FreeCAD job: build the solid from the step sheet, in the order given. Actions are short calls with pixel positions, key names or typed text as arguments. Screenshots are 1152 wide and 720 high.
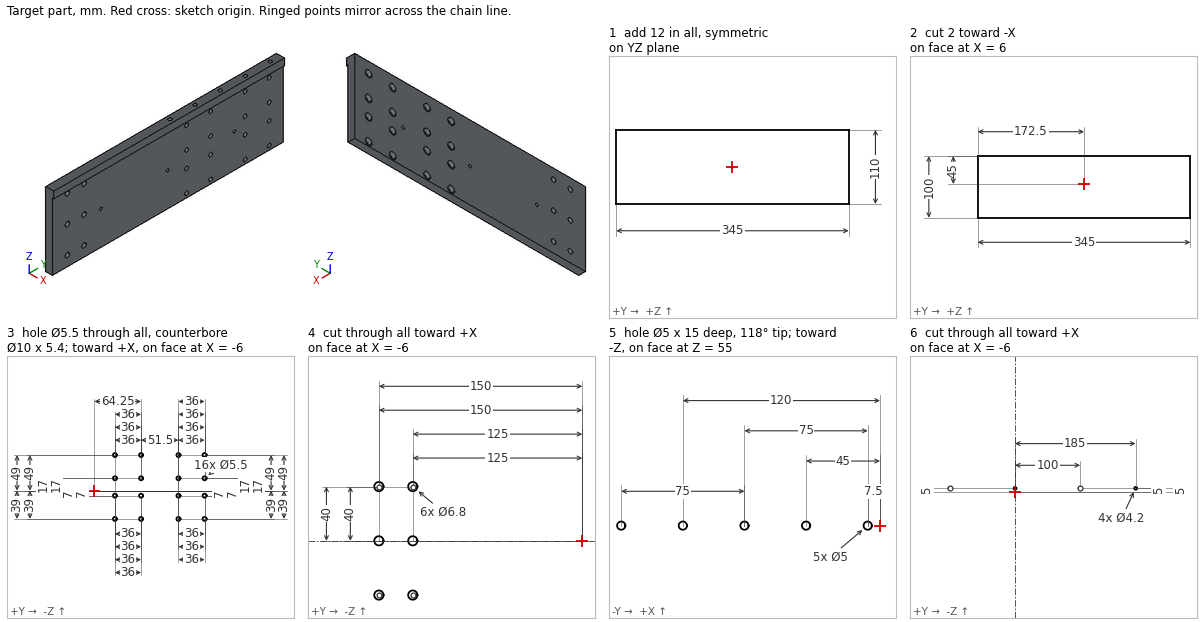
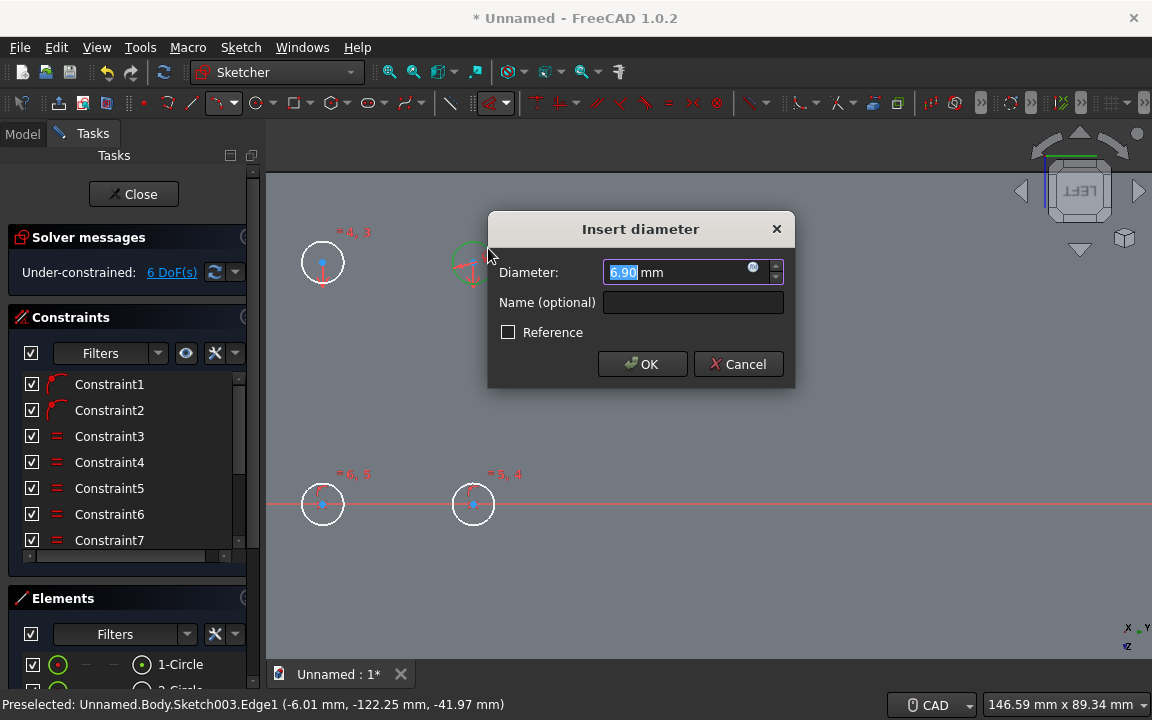
text(6.8)
key(Return)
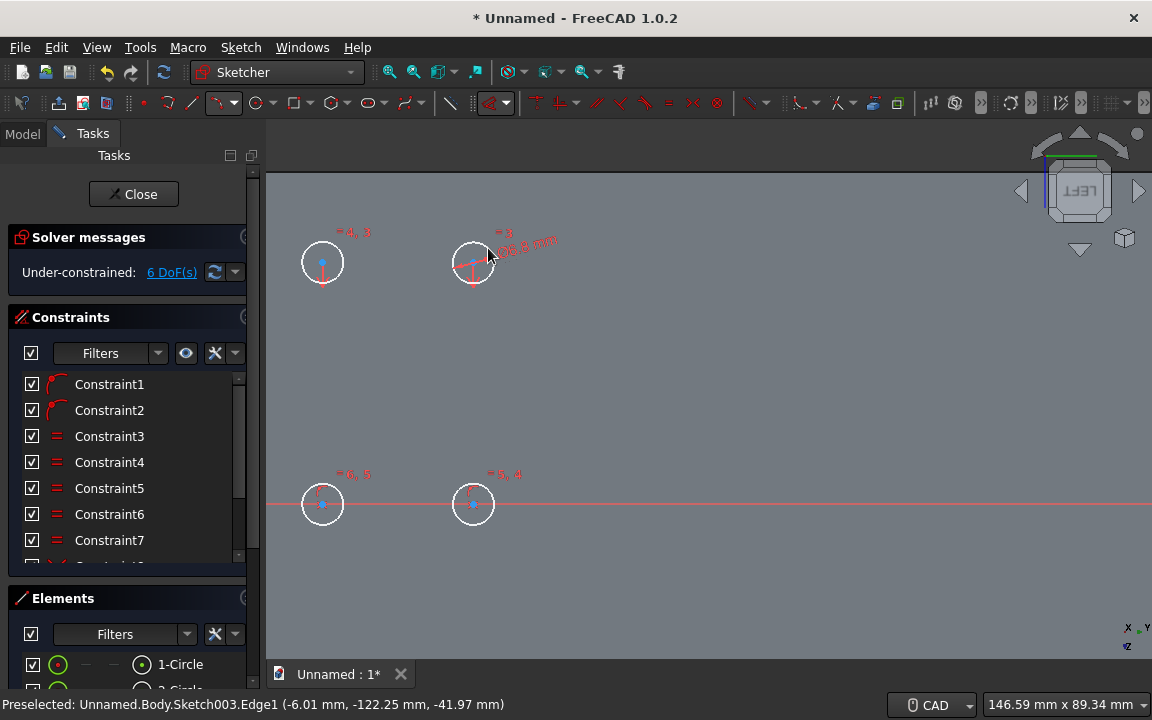
click(473, 263)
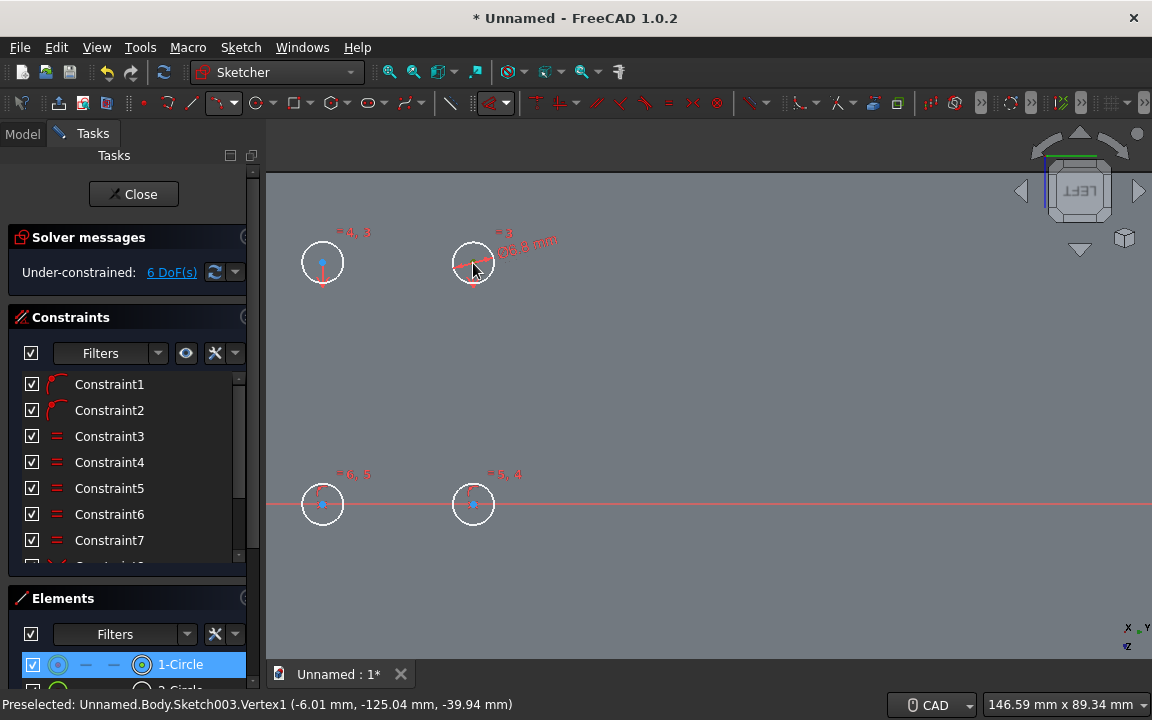
key(i)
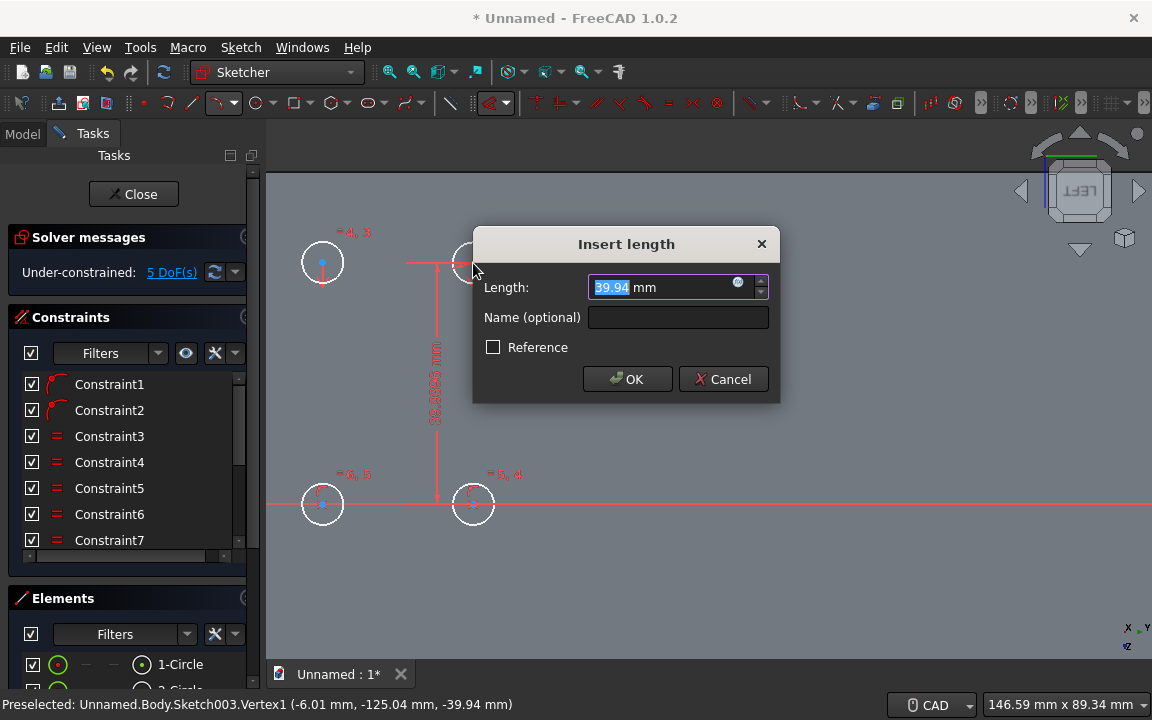
text(40)
key(Return)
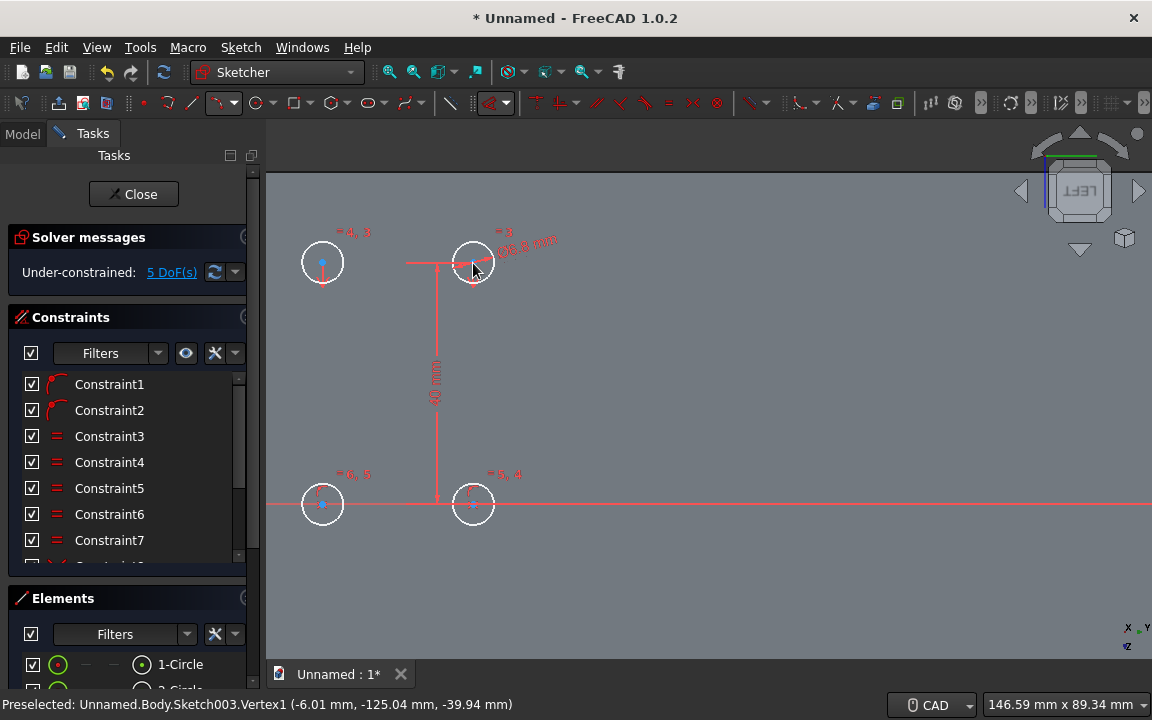
click(323, 262)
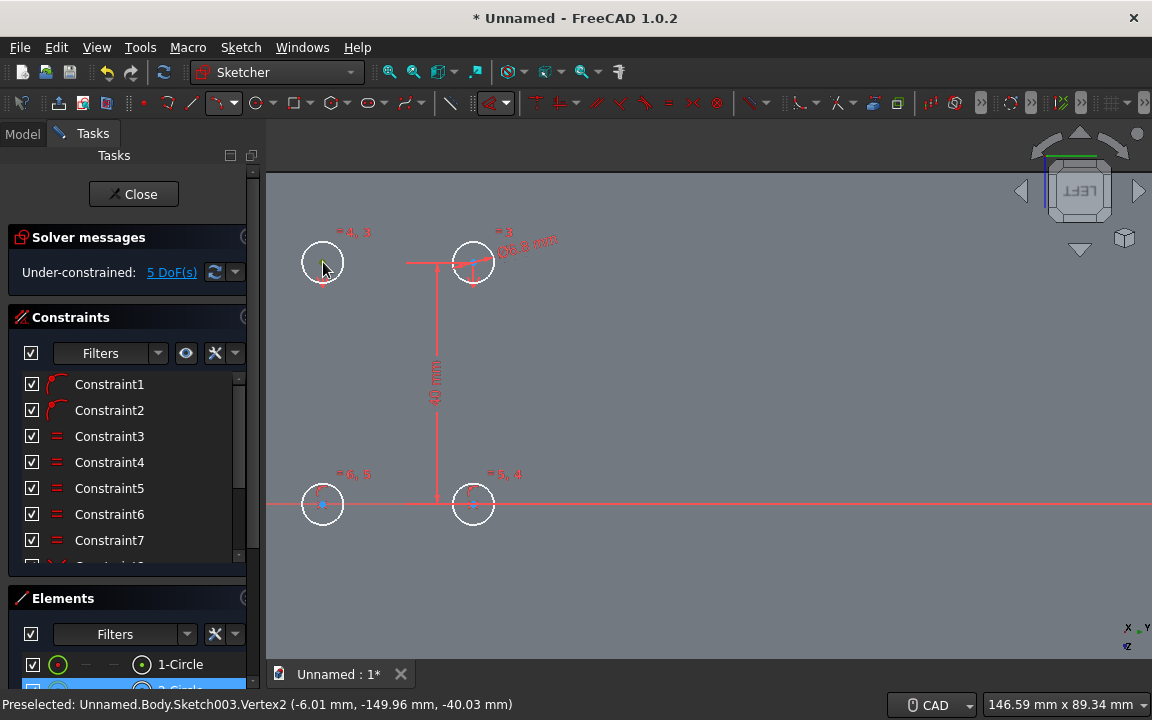
key(i)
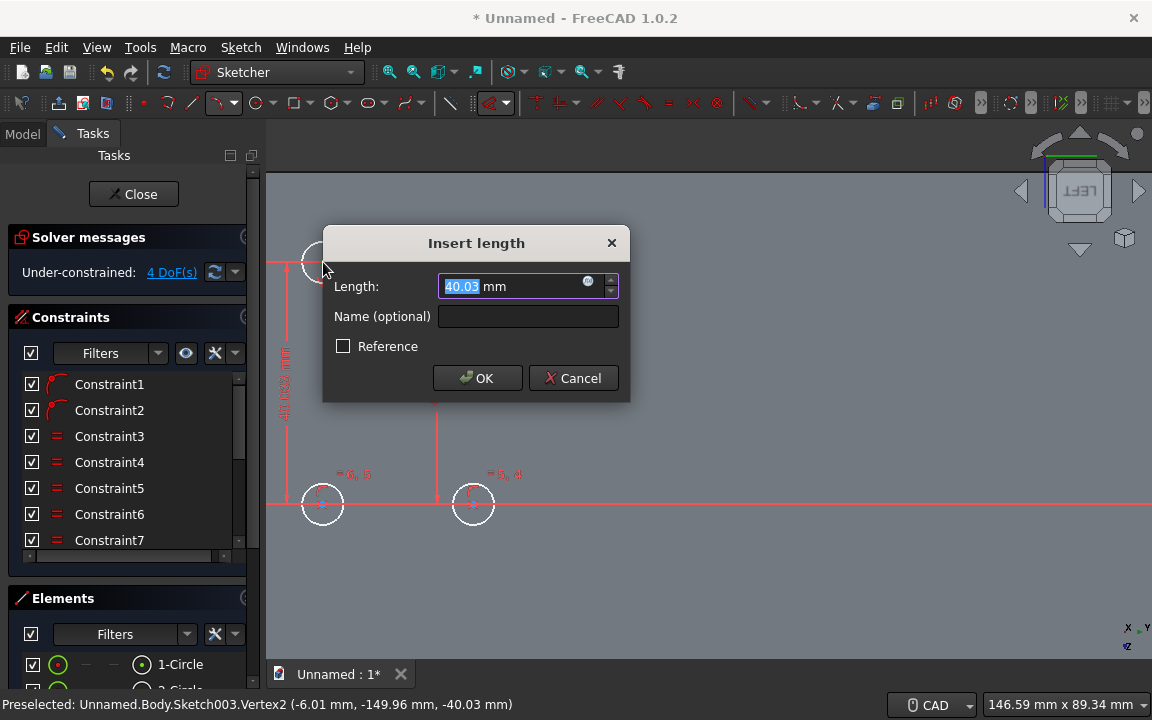
text(40)
key(Return)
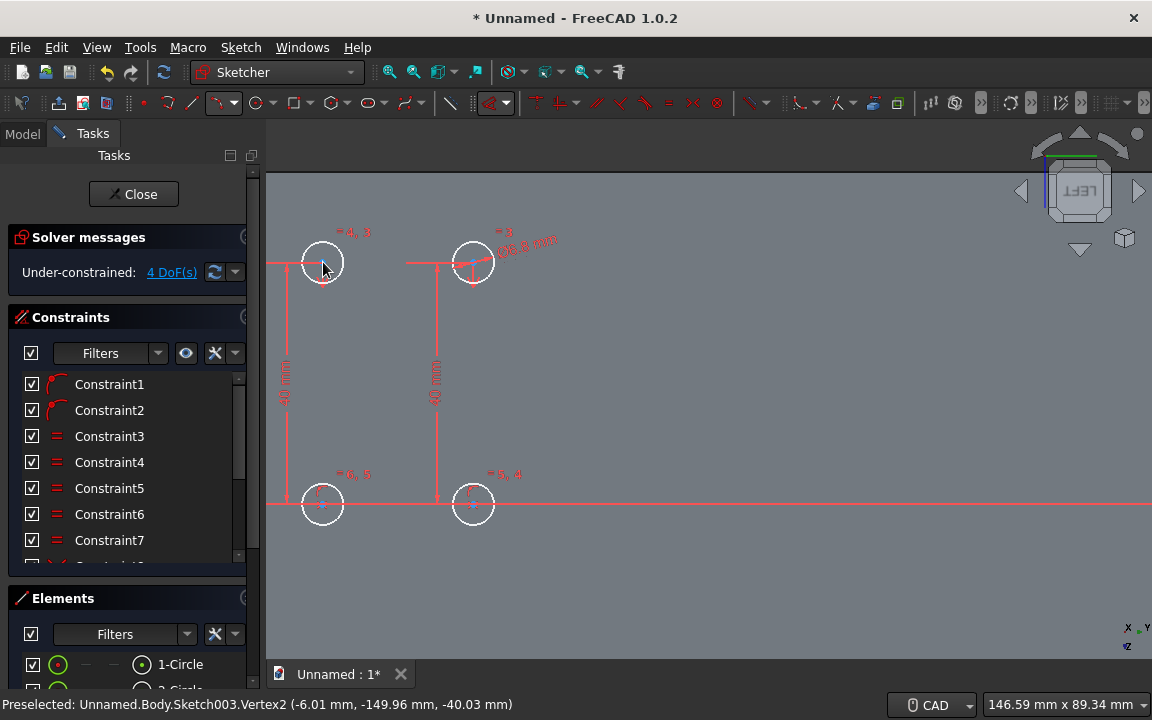
click(473, 263)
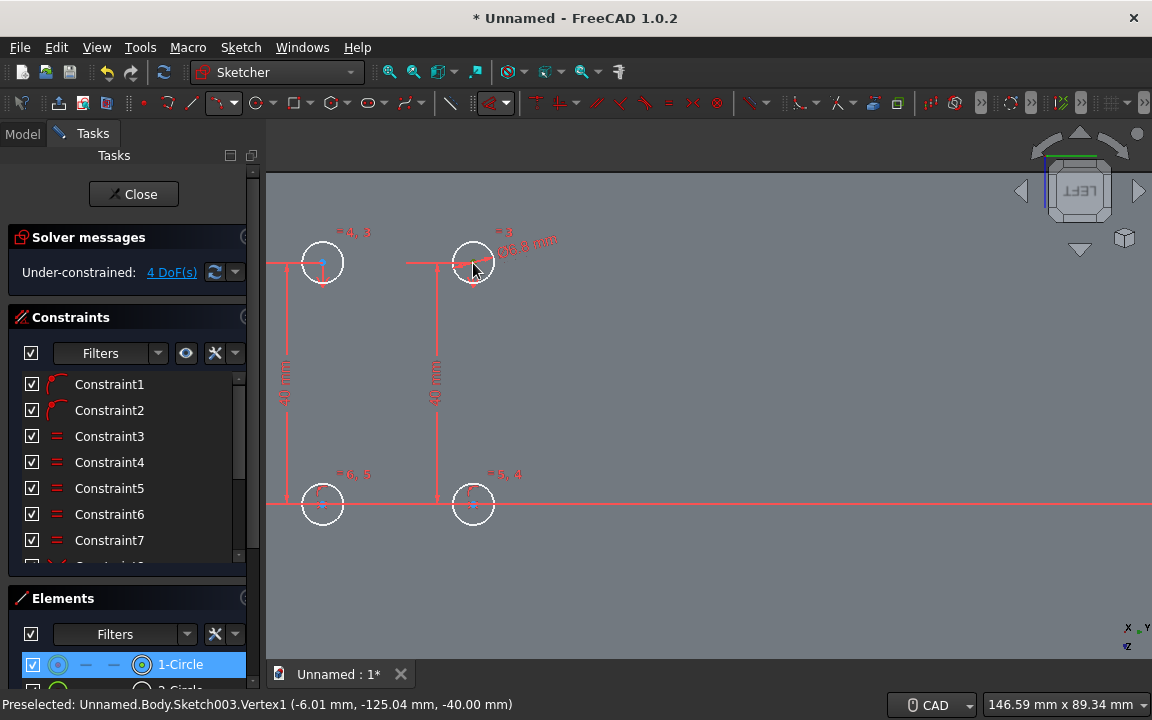
key(l)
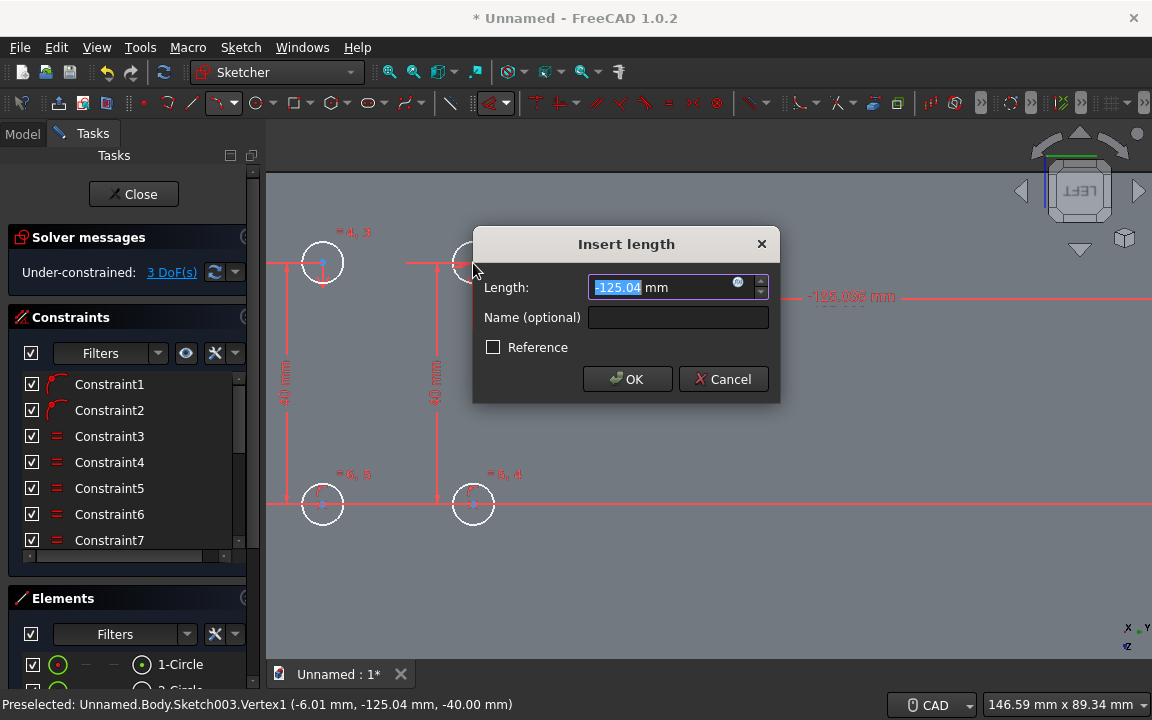
text(-125)
key(Return)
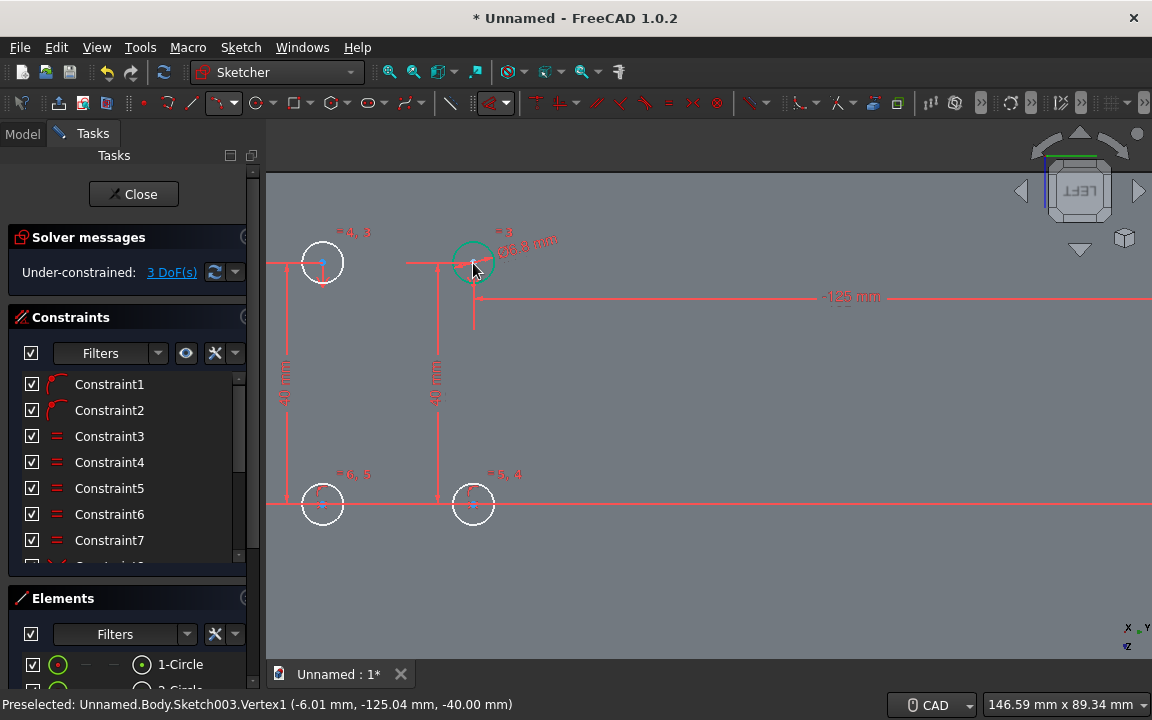
click(323, 263)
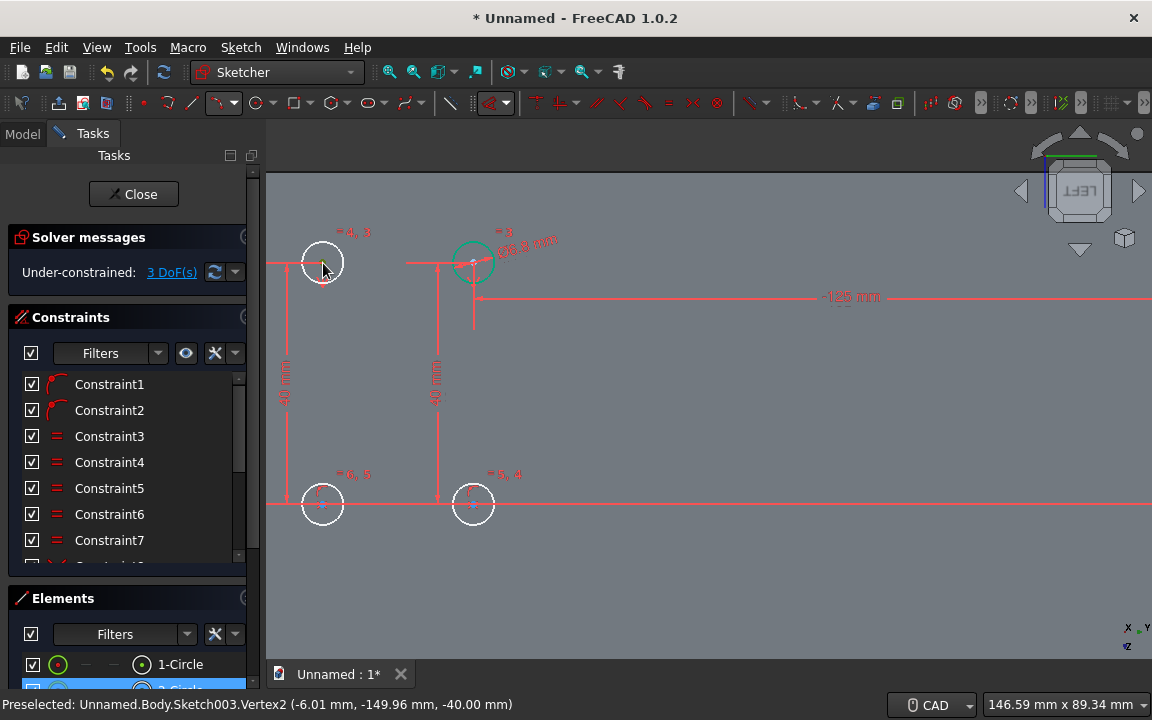
key(l)